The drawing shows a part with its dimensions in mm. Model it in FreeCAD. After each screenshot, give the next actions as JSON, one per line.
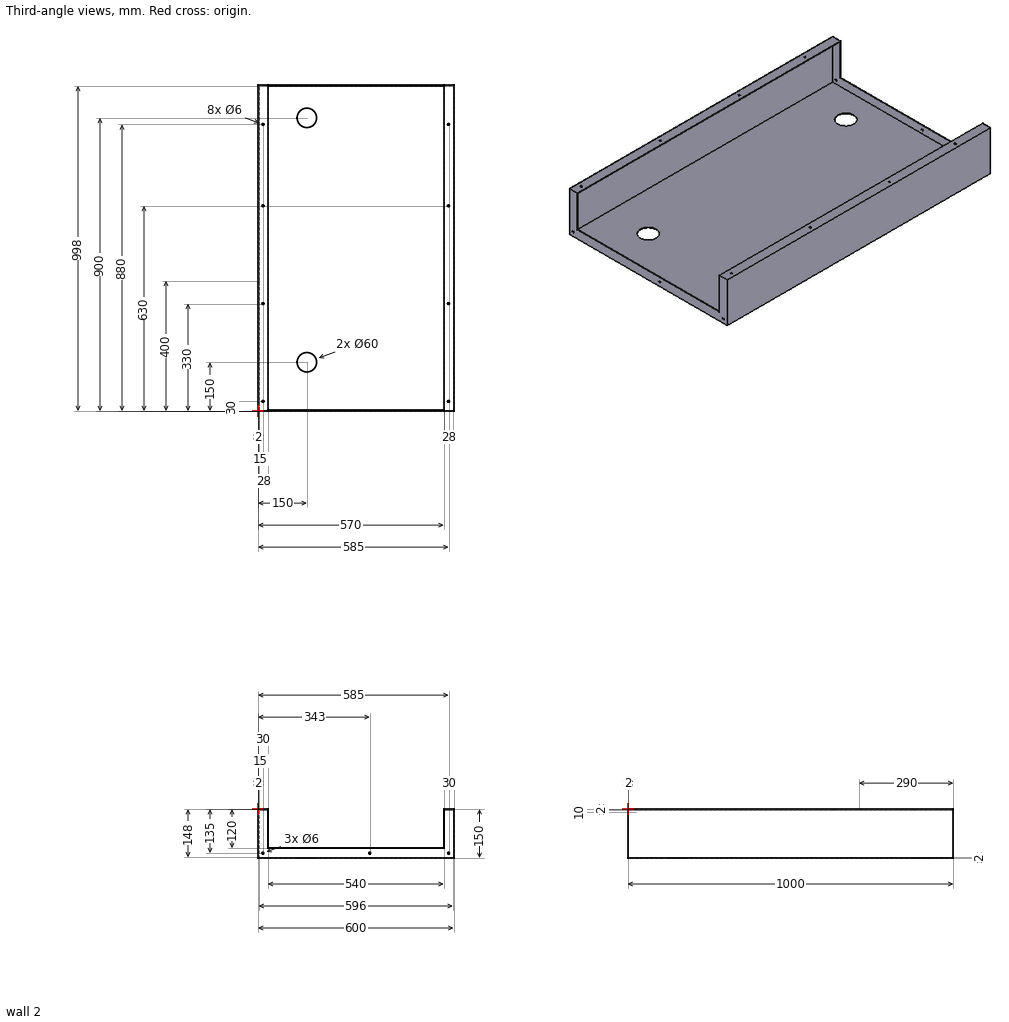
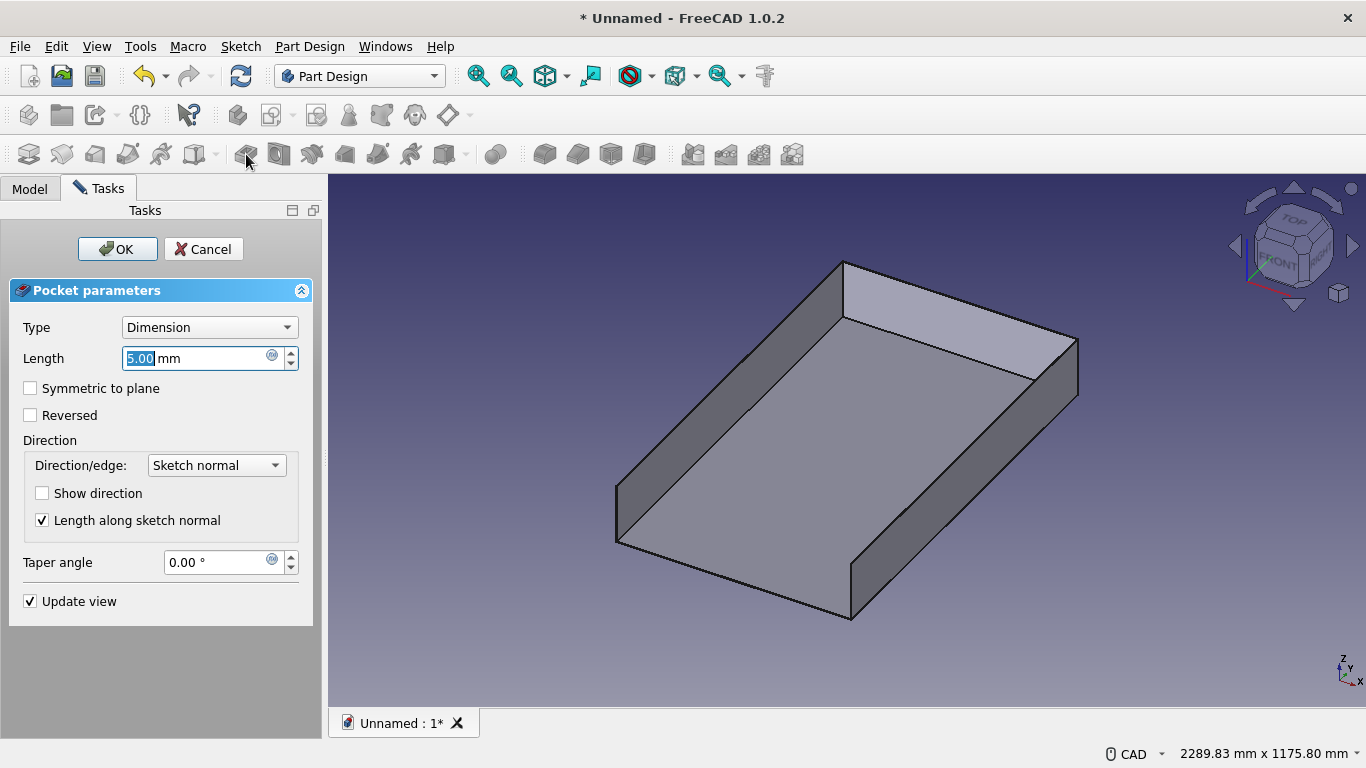
{"action": "type", "text": "400"}
{"action": "key", "text": "Tab"}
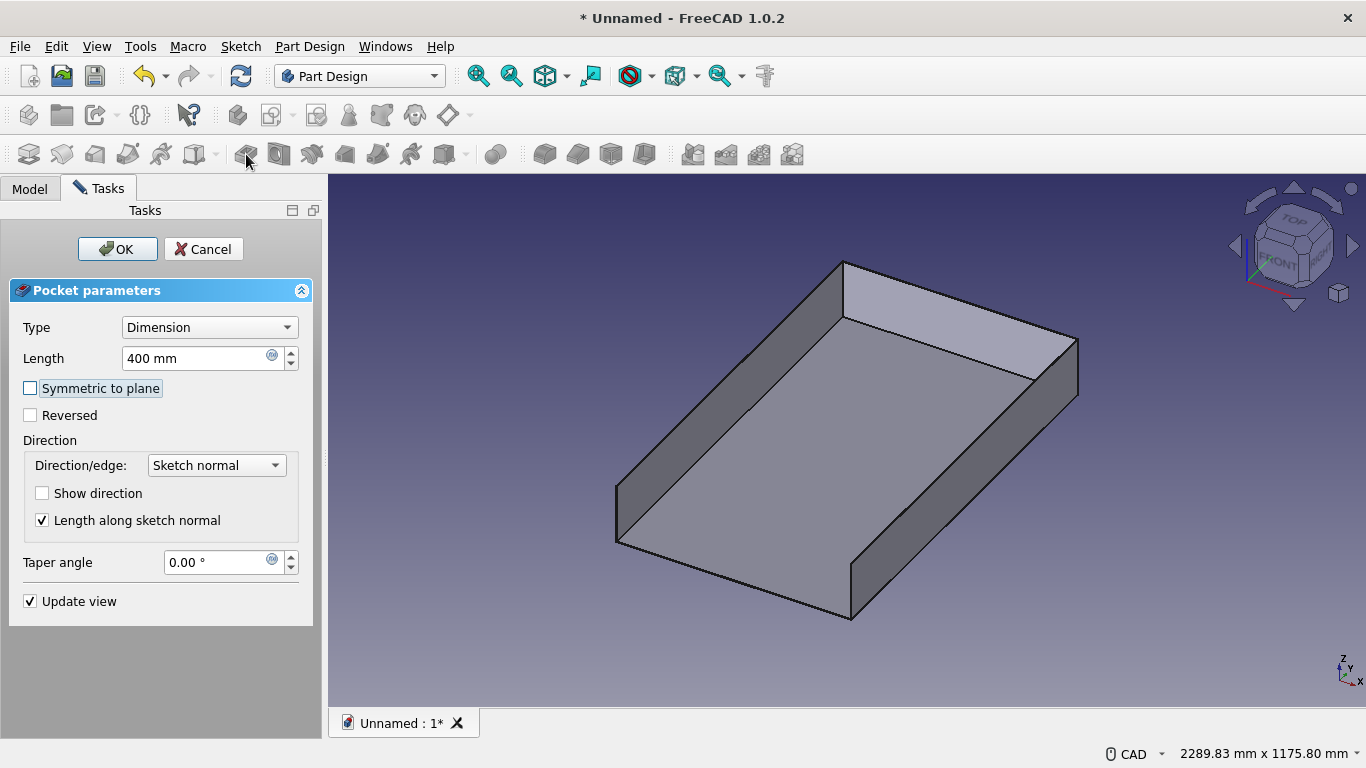
{"action": "left_click", "coordinate": [118, 249]}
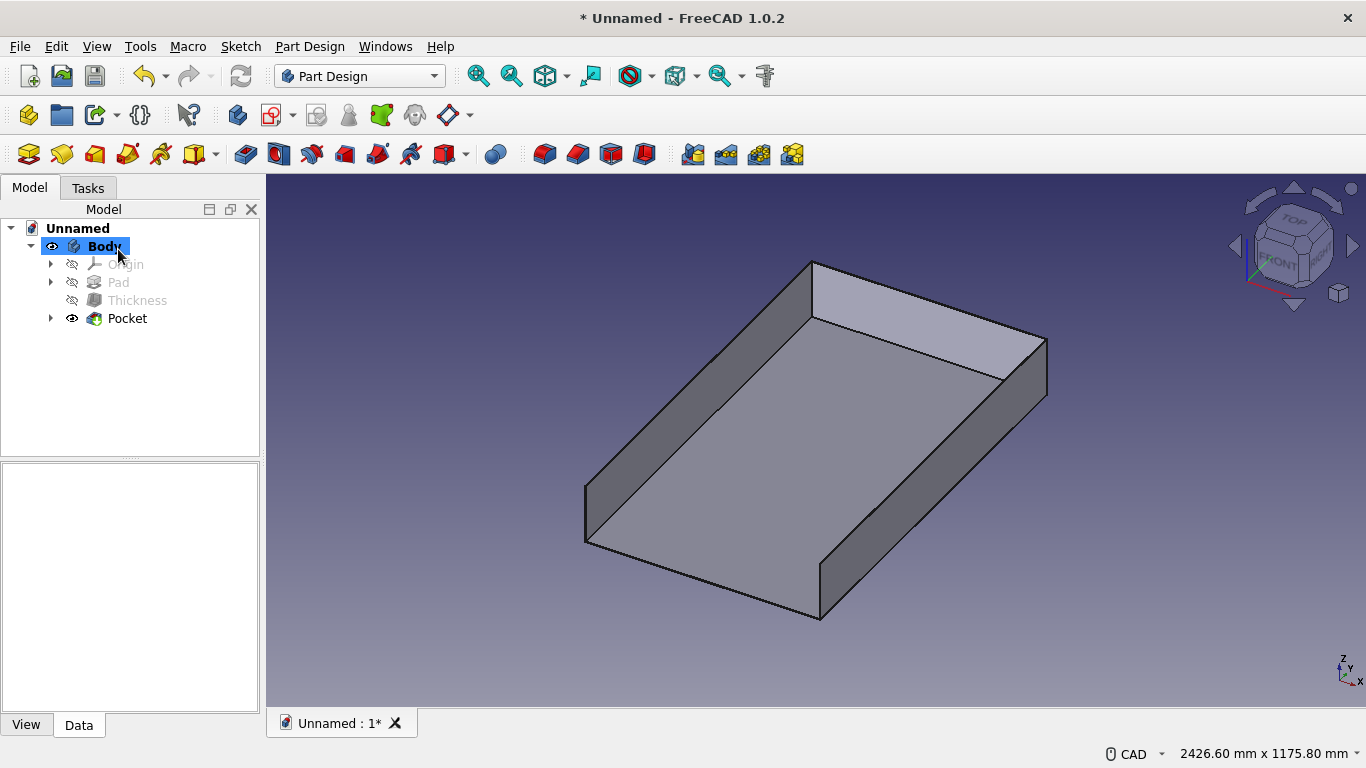
{"action": "scroll", "coordinate": [890, 286], "scroll_direction": "up", "scroll_amount": 15}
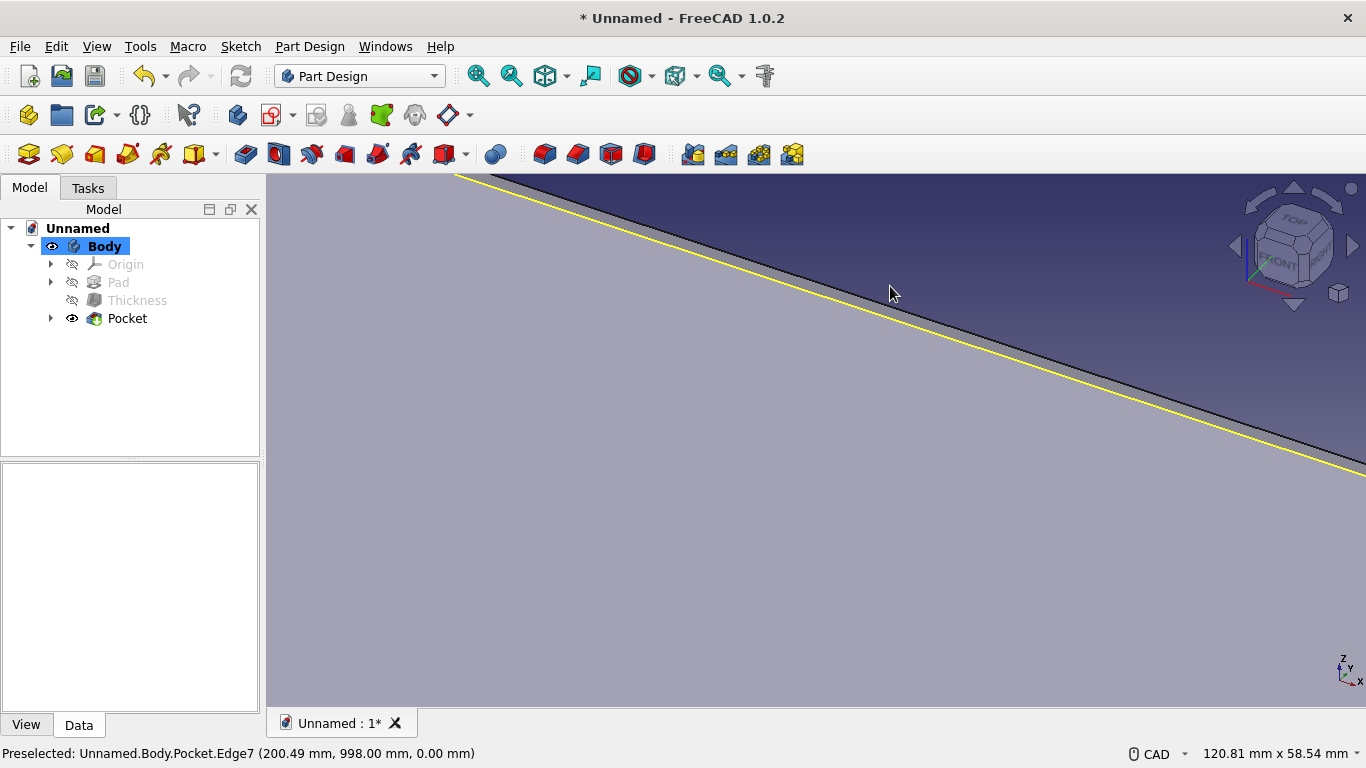
{"action": "scroll", "coordinate": [874, 308], "scroll_direction": "up", "scroll_amount": 4}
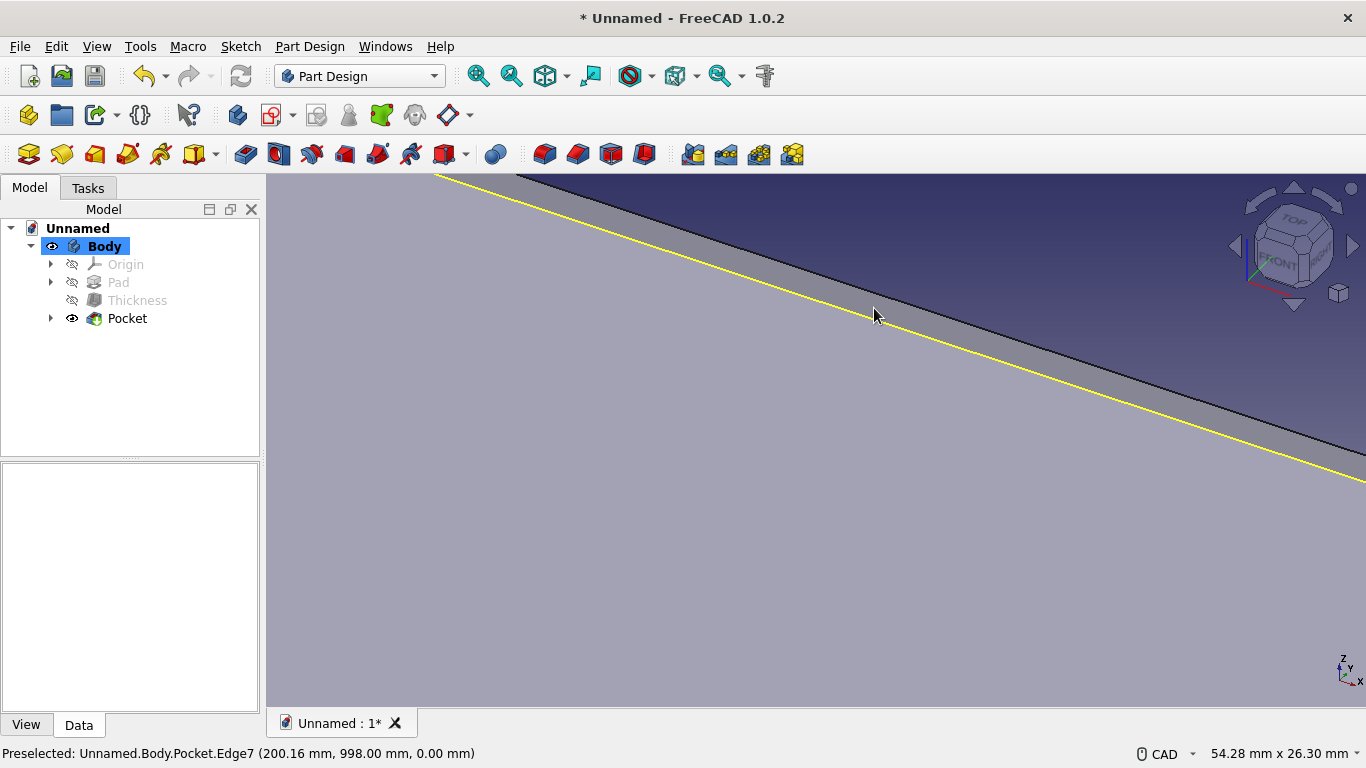
{"action": "left_click", "coordinate": [479, 76]}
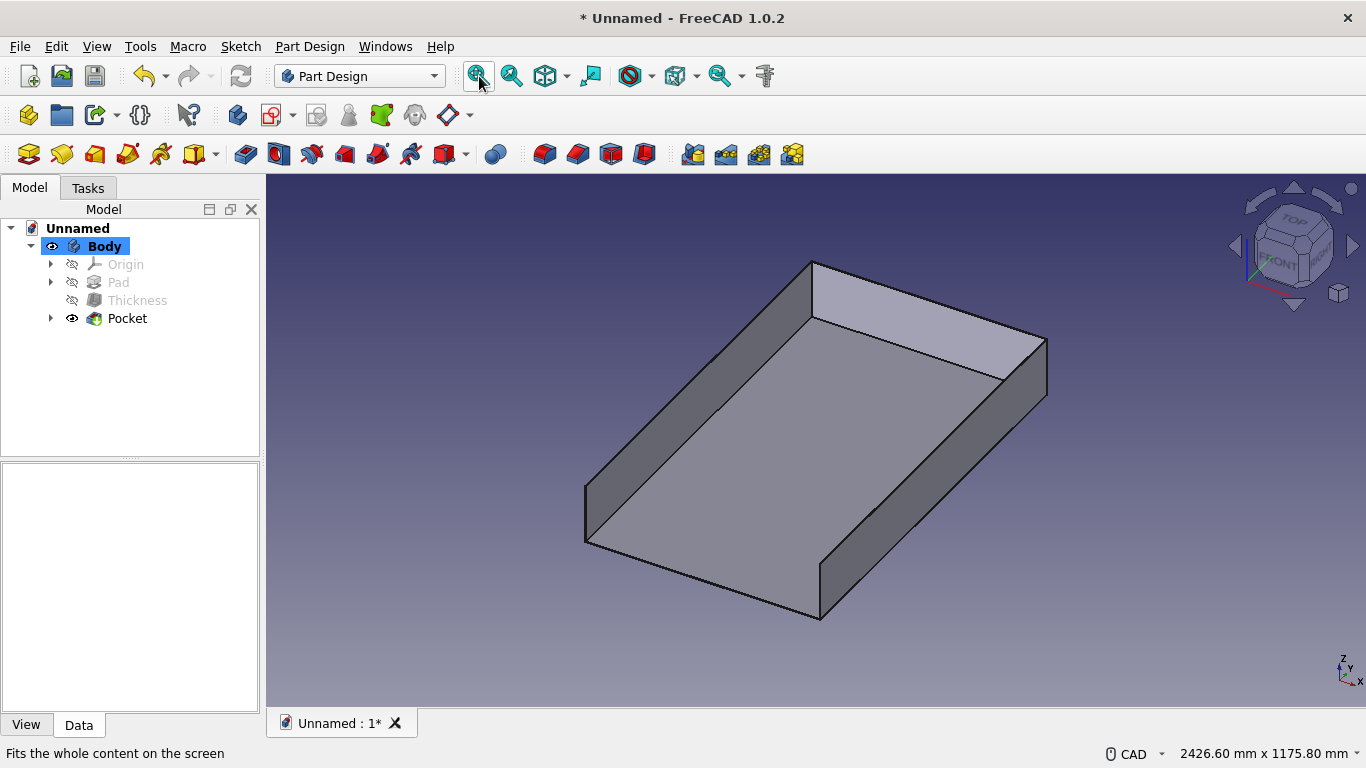
{"action": "key", "text": "0"}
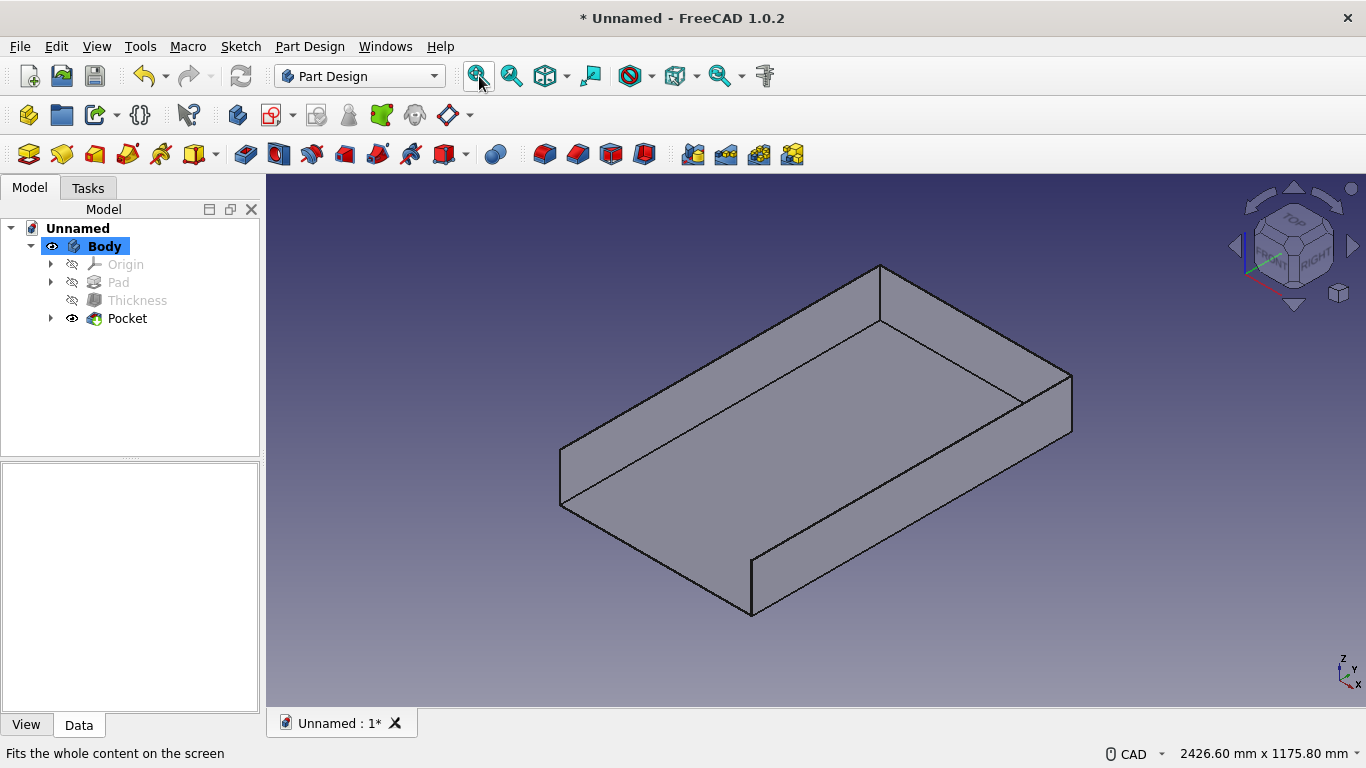
{"action": "scroll", "coordinate": [944, 301], "scroll_direction": "up", "scroll_amount": 15}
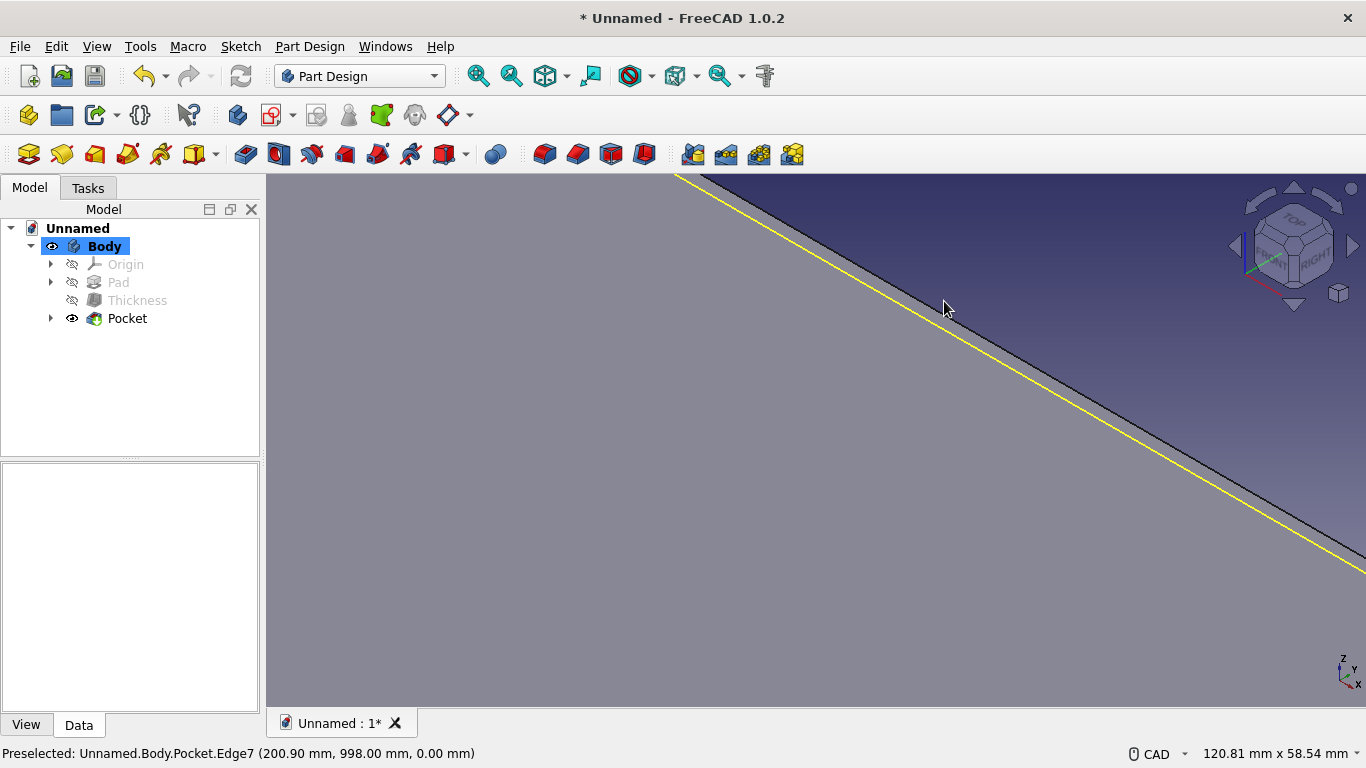
{"action": "scroll", "coordinate": [928, 315], "scroll_direction": "up", "scroll_amount": 4}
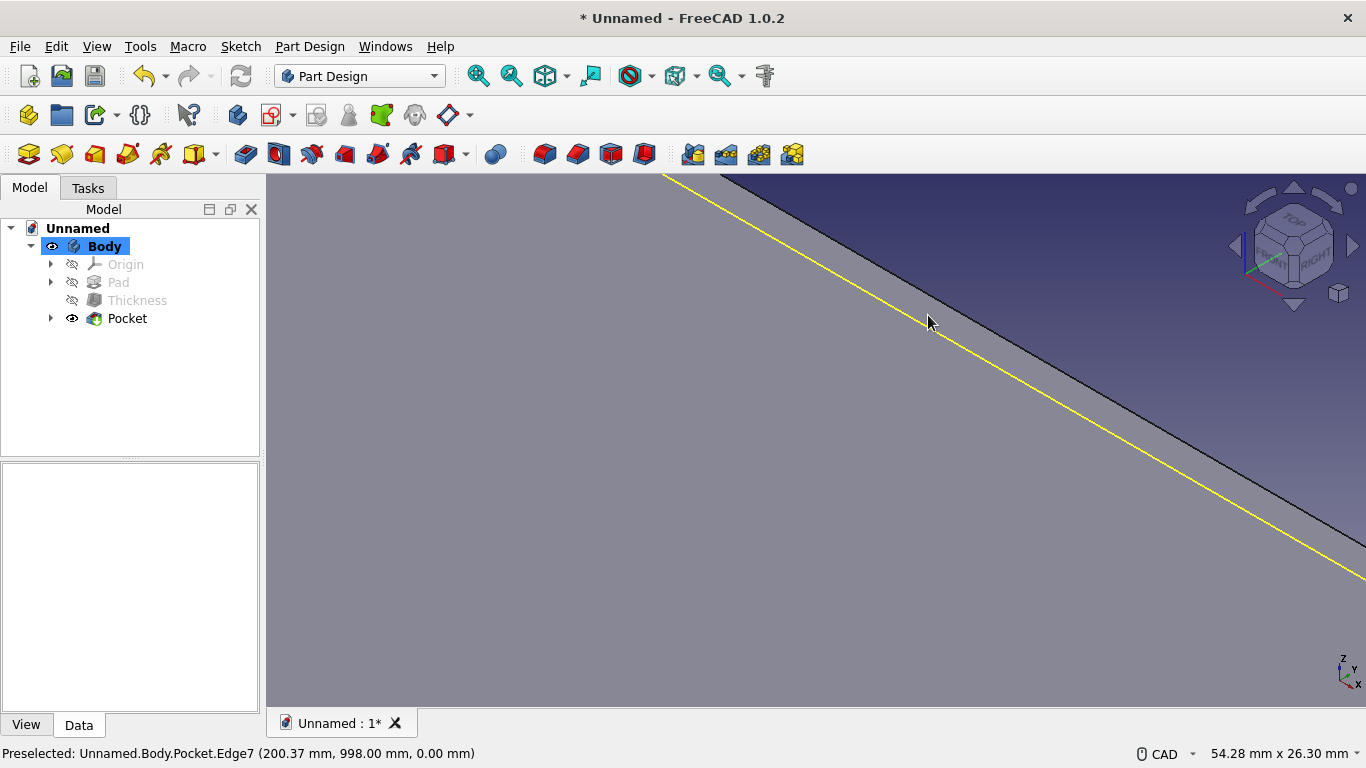
{"action": "left_click", "coordinate": [927, 315]}